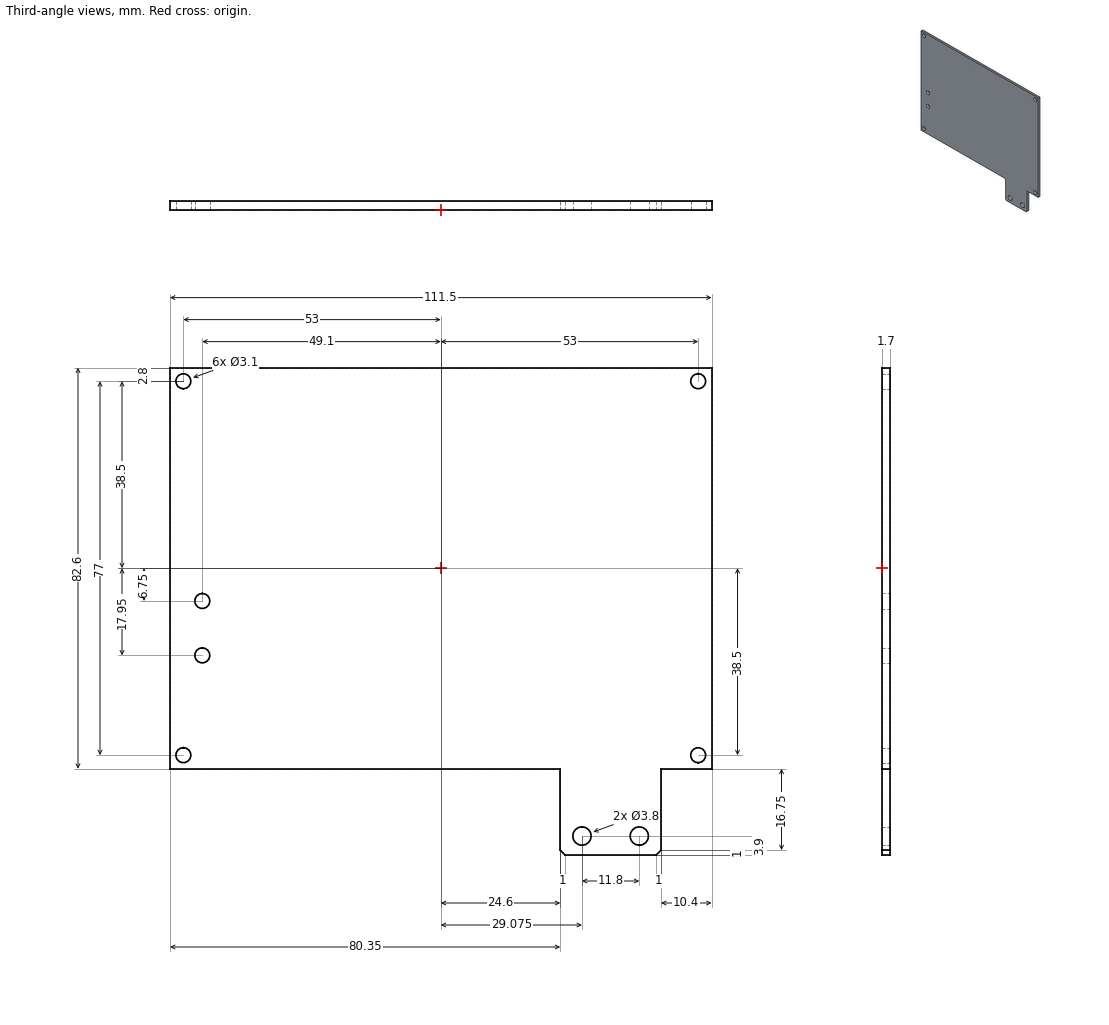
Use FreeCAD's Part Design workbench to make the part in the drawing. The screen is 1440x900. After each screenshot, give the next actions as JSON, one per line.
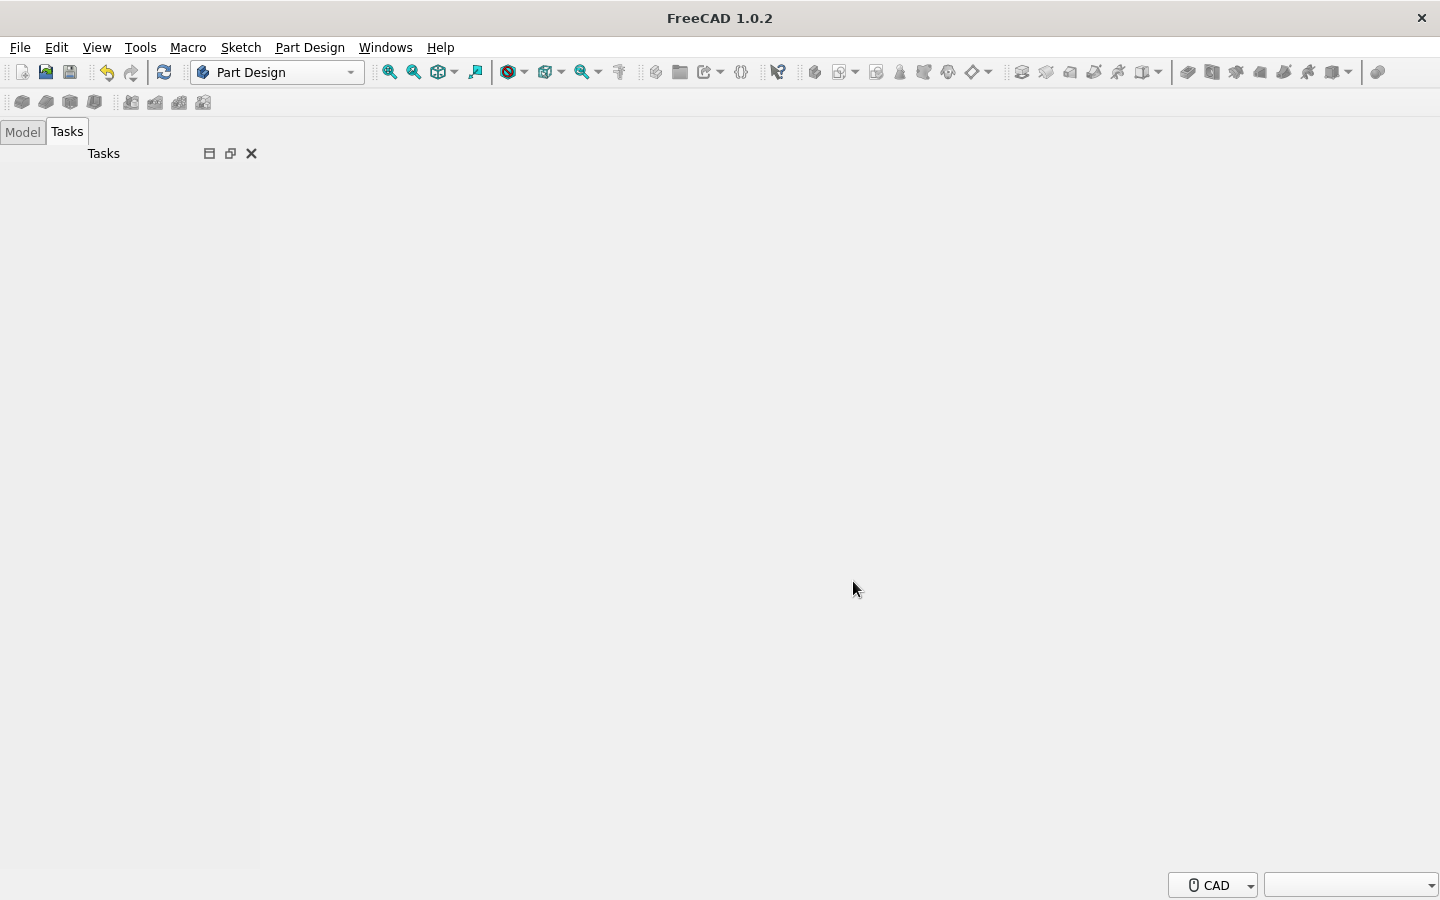
{"action": "key", "text": "ctrl+n"}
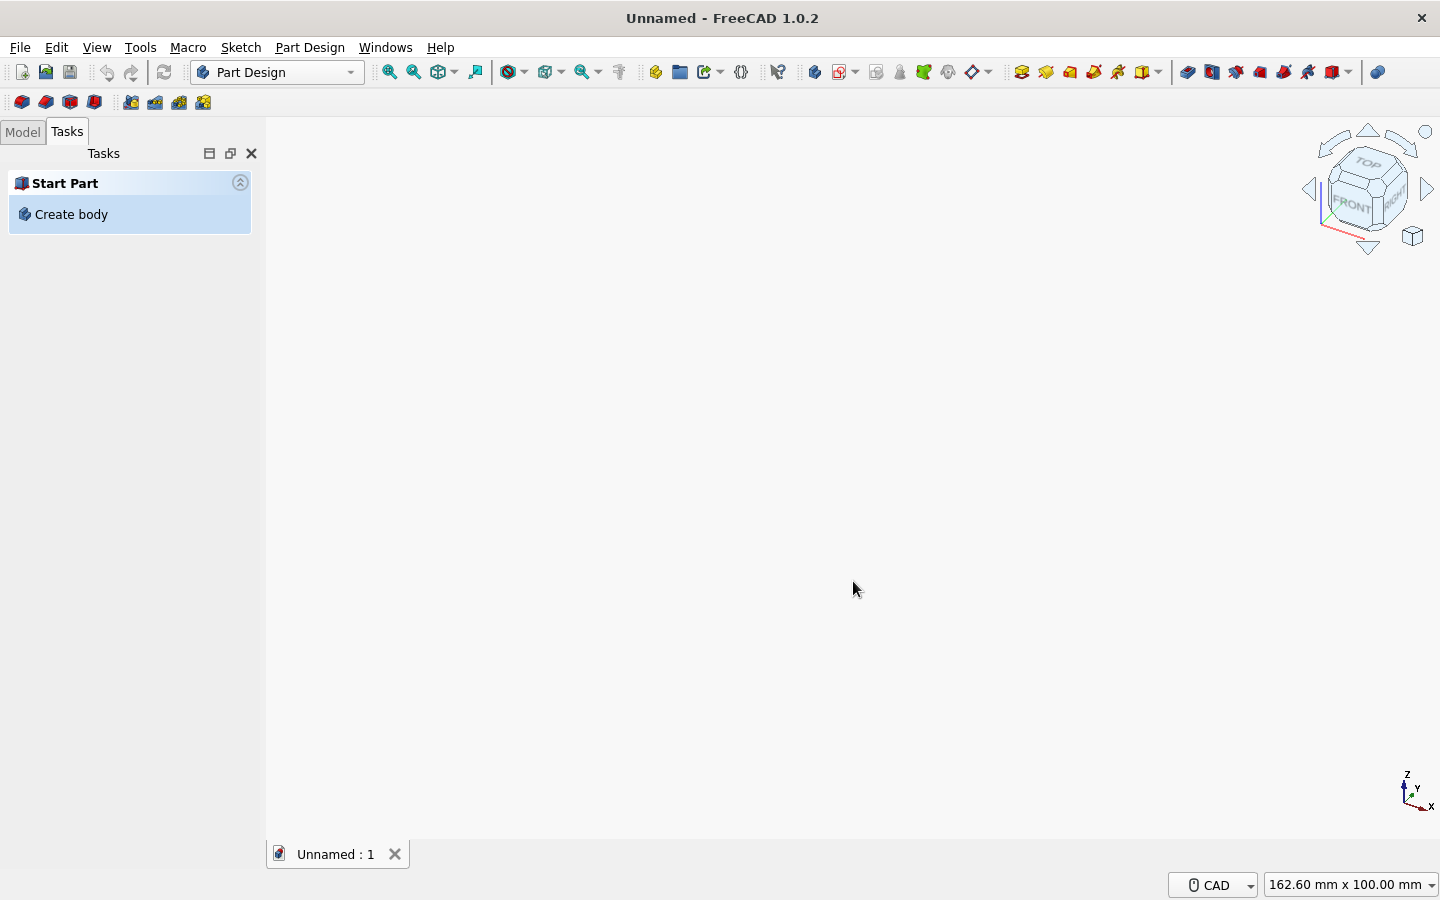
{"action": "left_click", "coordinate": [840, 72]}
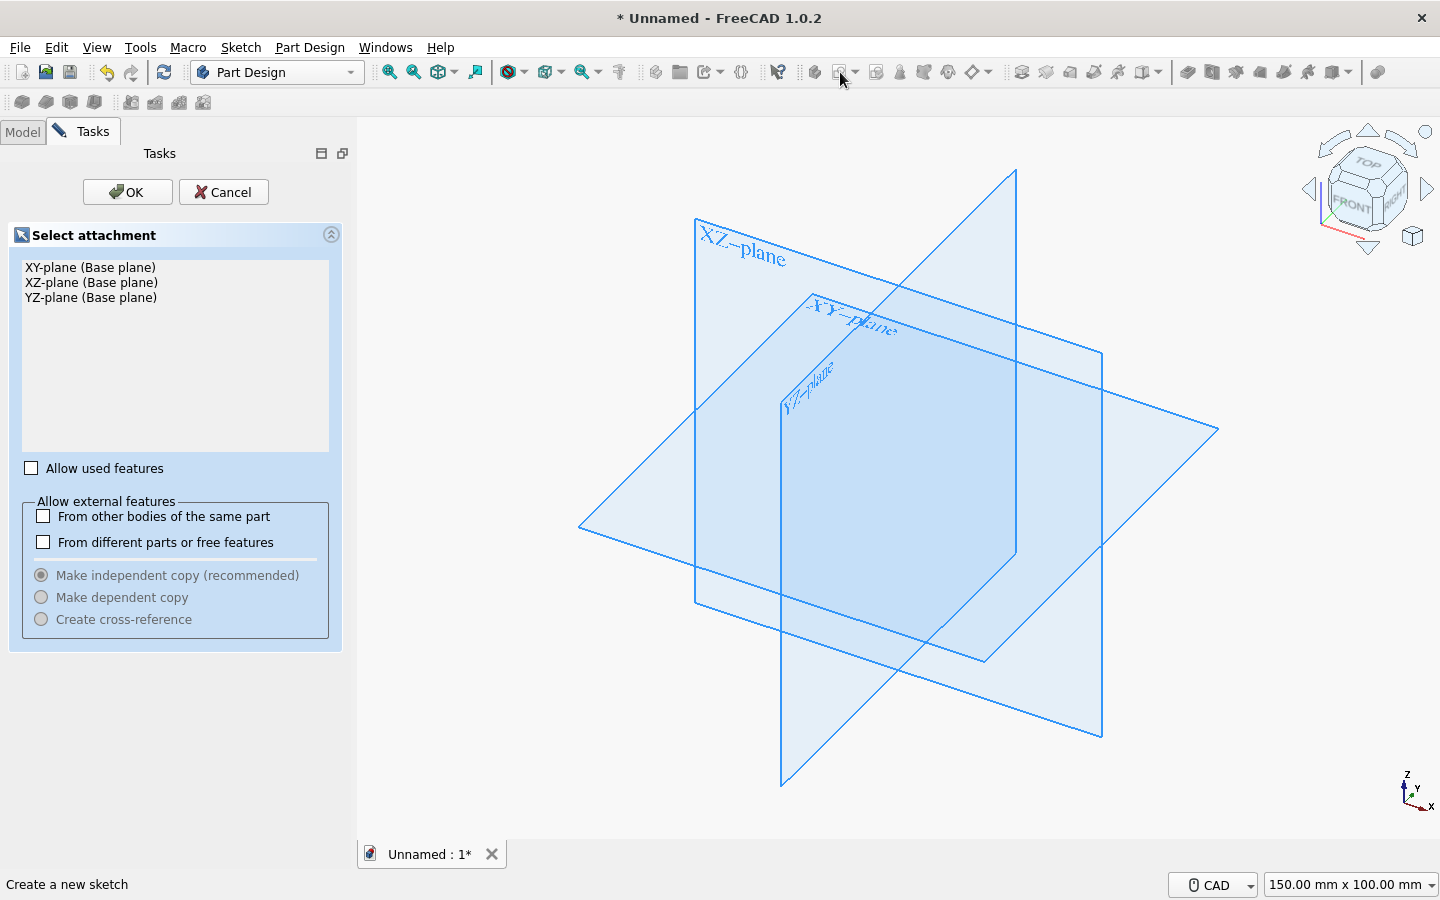
{"action": "left_click", "coordinate": [82, 282]}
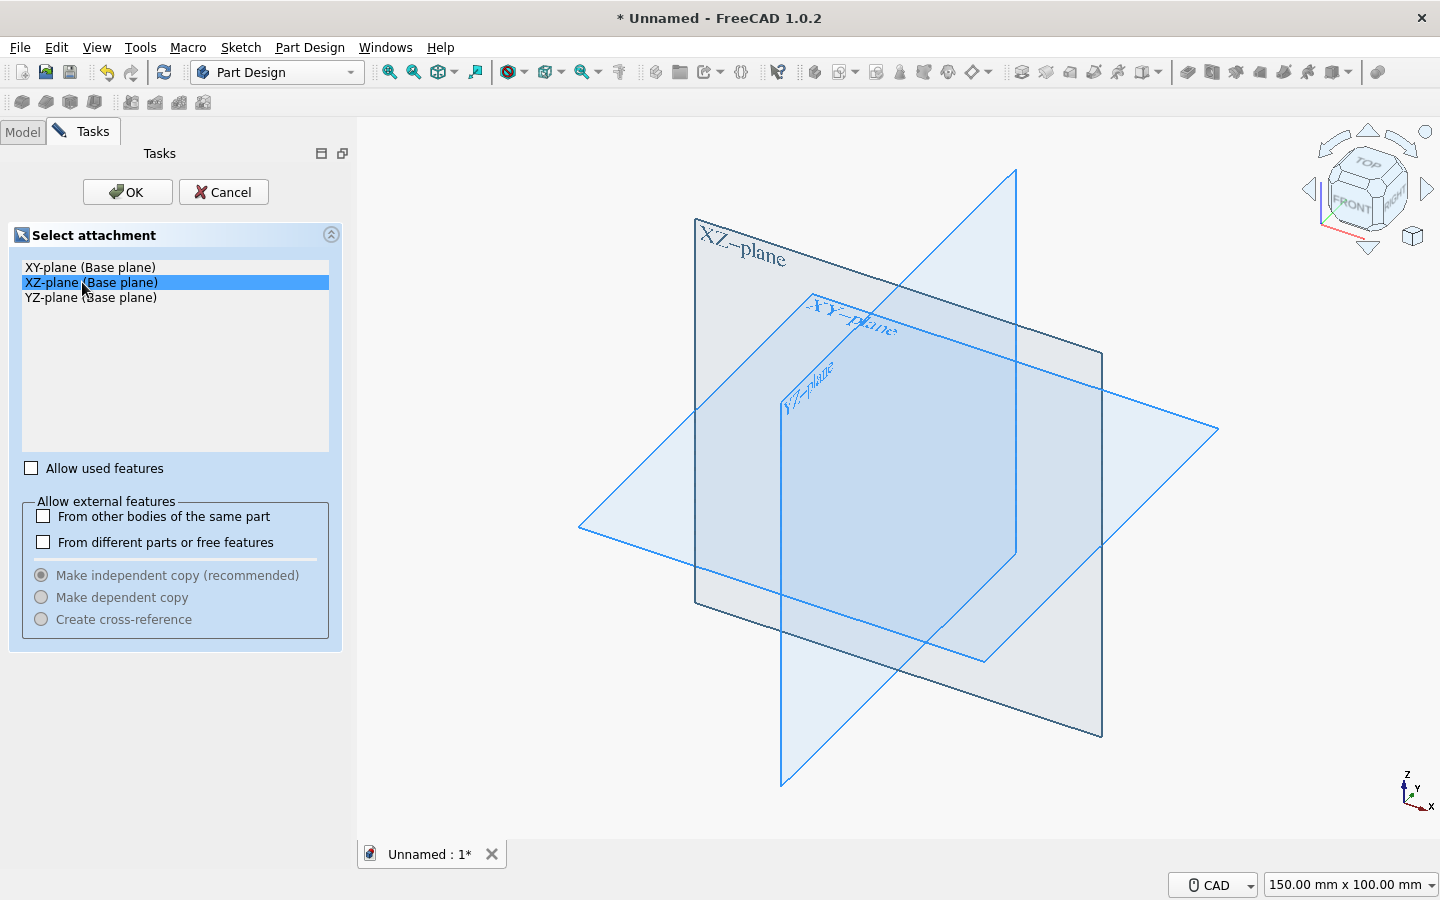
{"action": "left_click", "coordinate": [128, 192]}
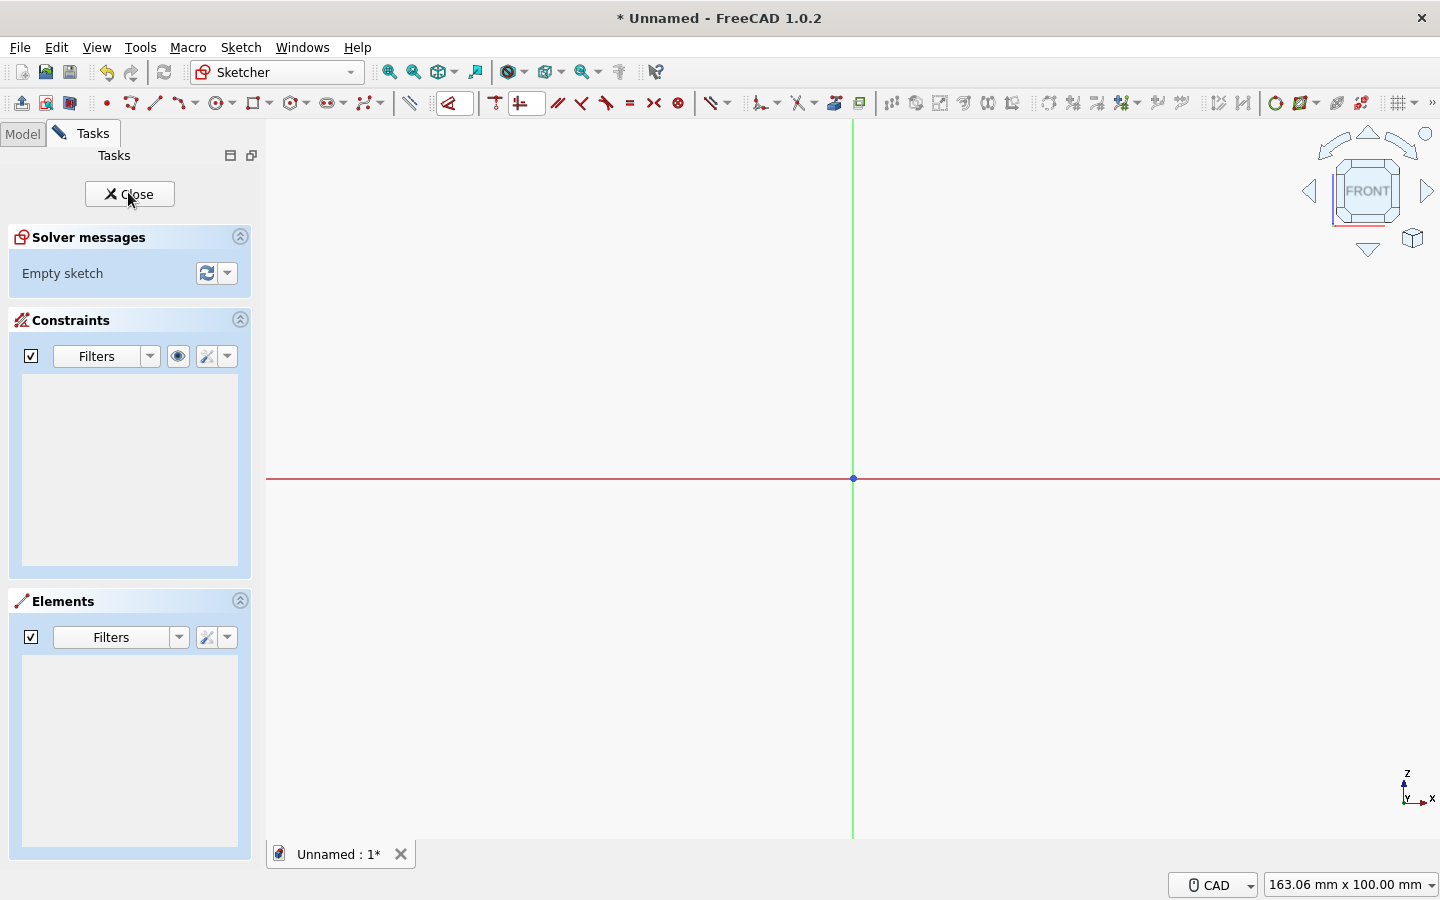
{"action": "scroll", "coordinate": [645, 349], "scroll_direction": "down", "scroll_amount": 2}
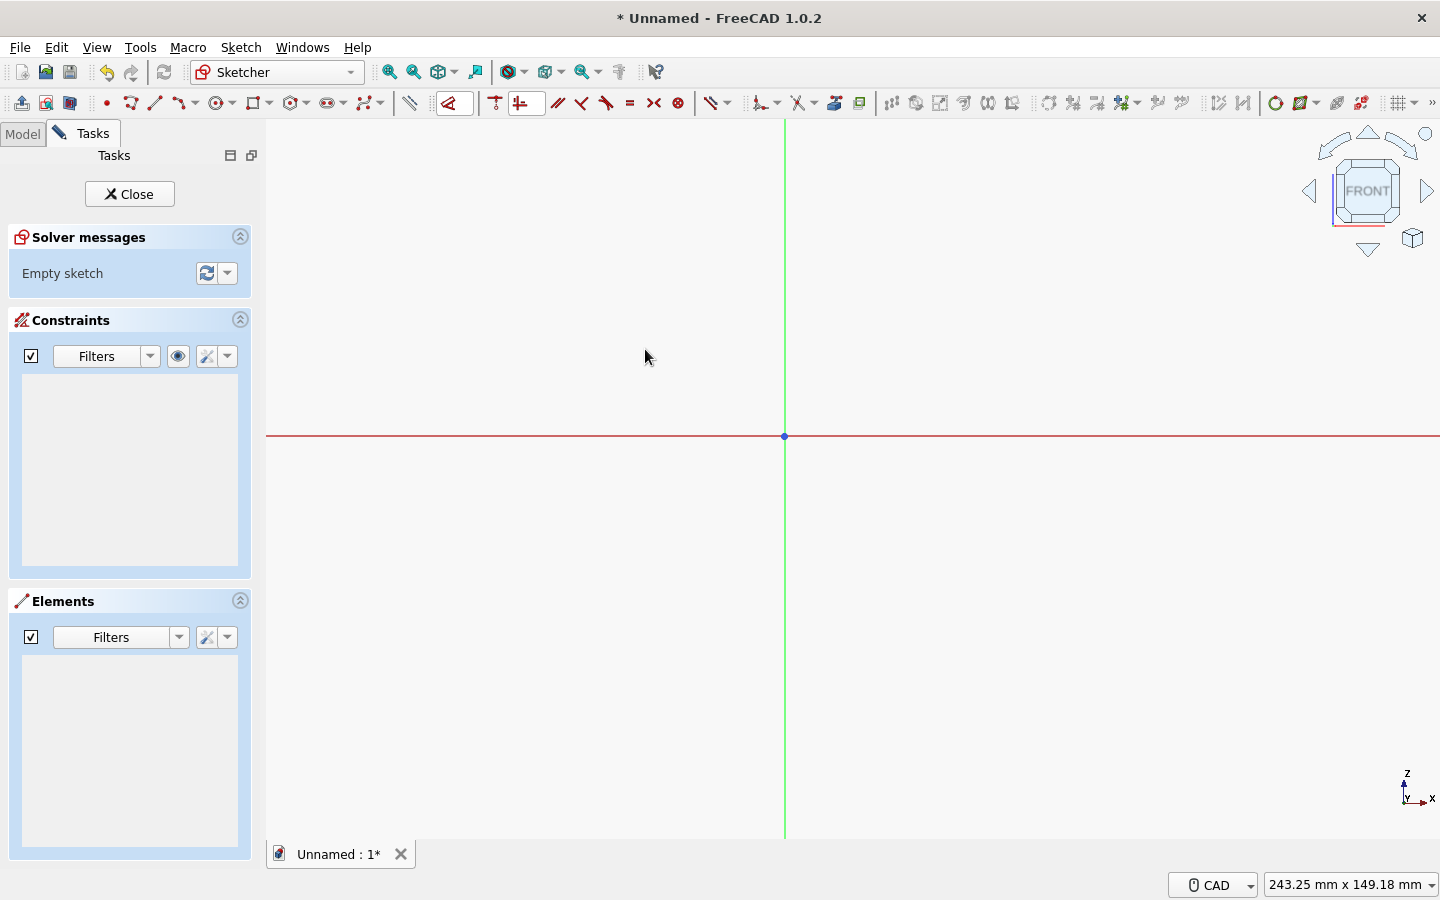
{"action": "key", "text": "g m"}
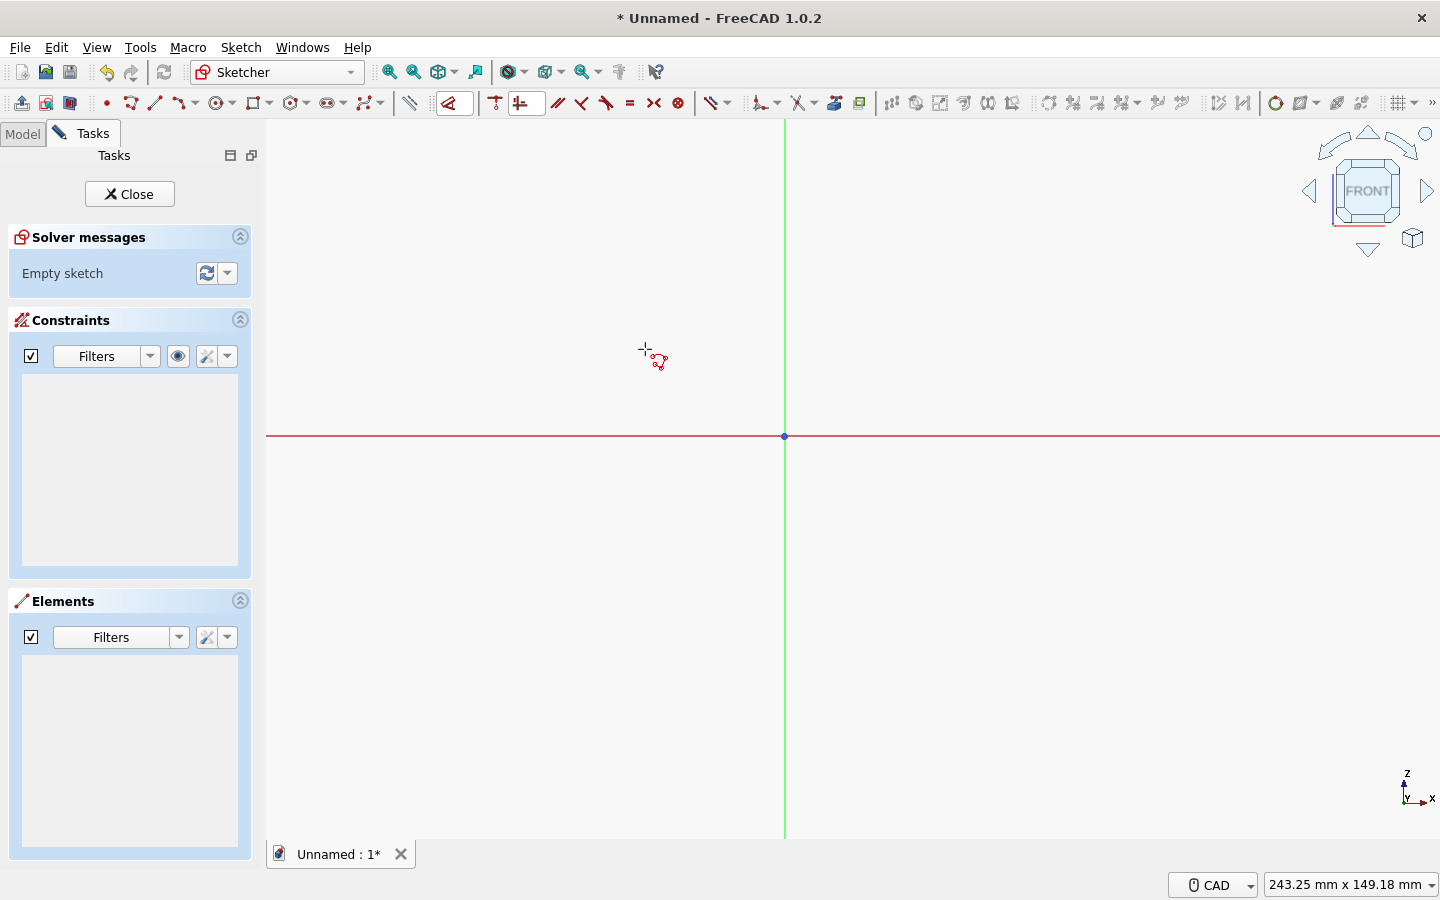
{"action": "left_click", "coordinate": [903, 636]}
{"action": "left_click", "coordinate": [515, 636]}
{"action": "left_click", "coordinate": [515, 237]}
{"action": "left_click", "coordinate": [1054, 237]}
{"action": "left_click", "coordinate": [1054, 636]}
{"action": "left_click", "coordinate": [1003, 636]}
{"action": "left_click", "coordinate": [1003, 716]}